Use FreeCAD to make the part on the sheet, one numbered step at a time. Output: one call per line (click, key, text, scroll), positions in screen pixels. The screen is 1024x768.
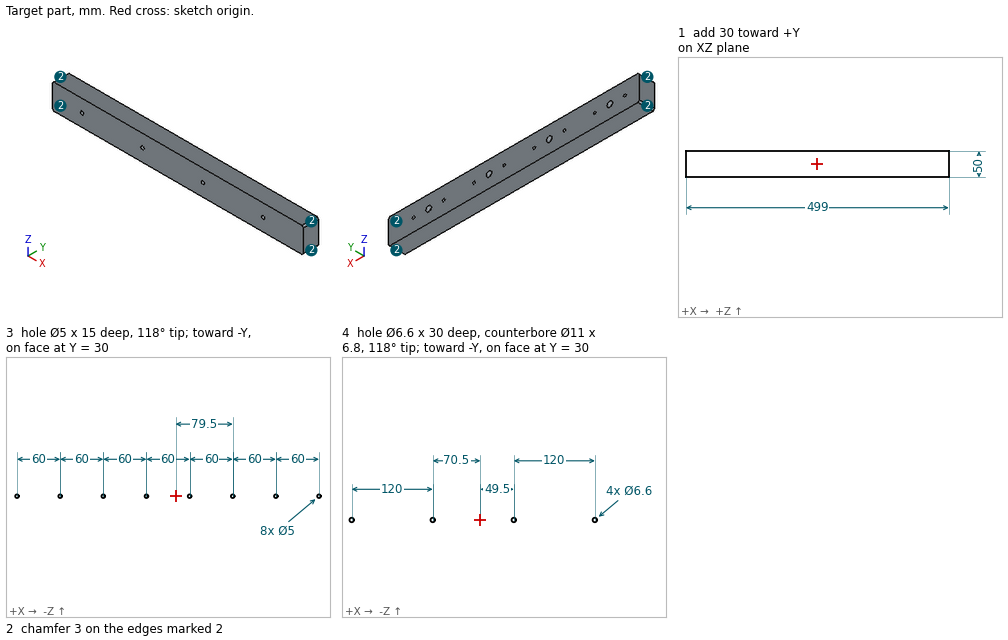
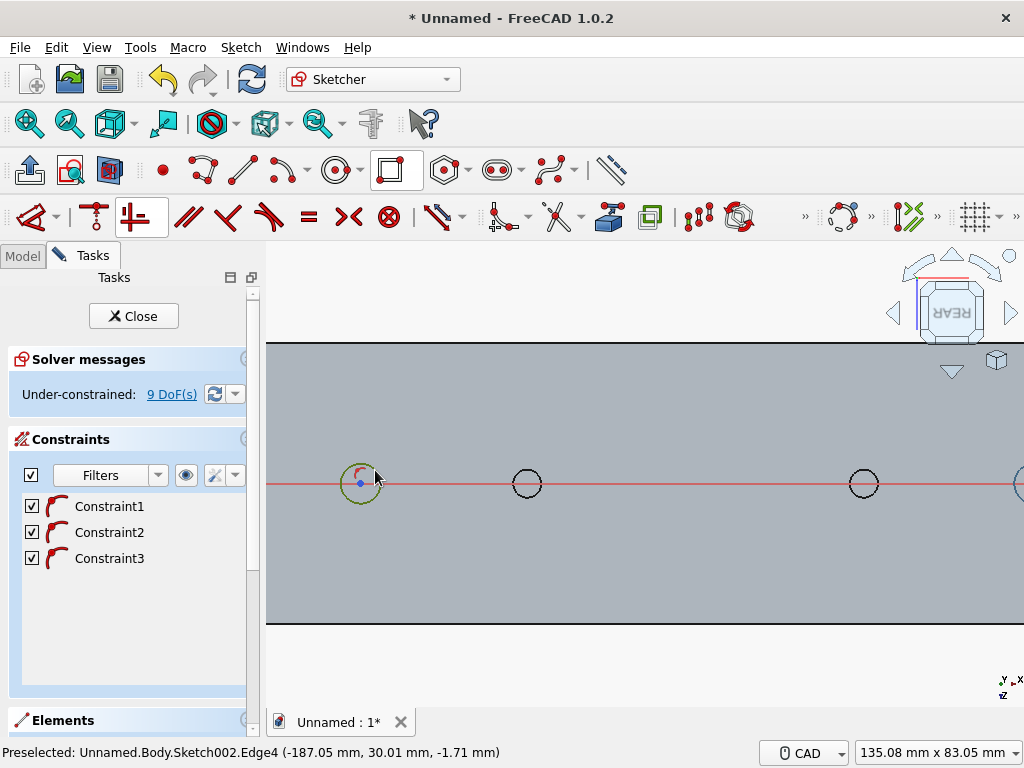
click(310, 218)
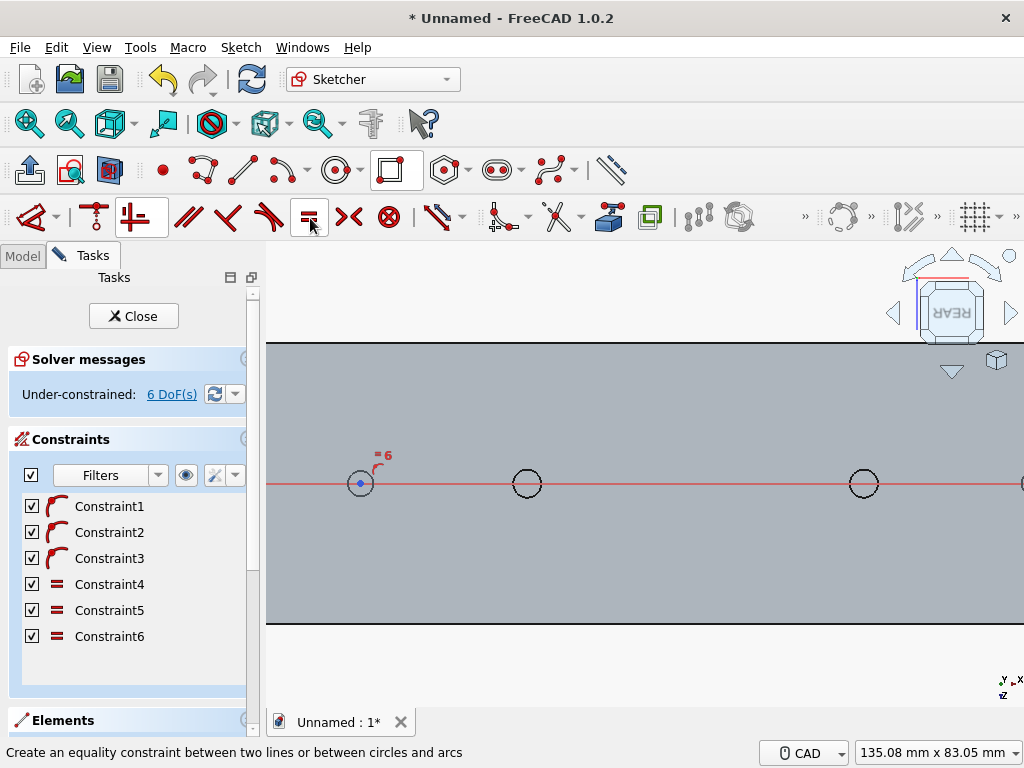
scroll(376, 472, down, 8)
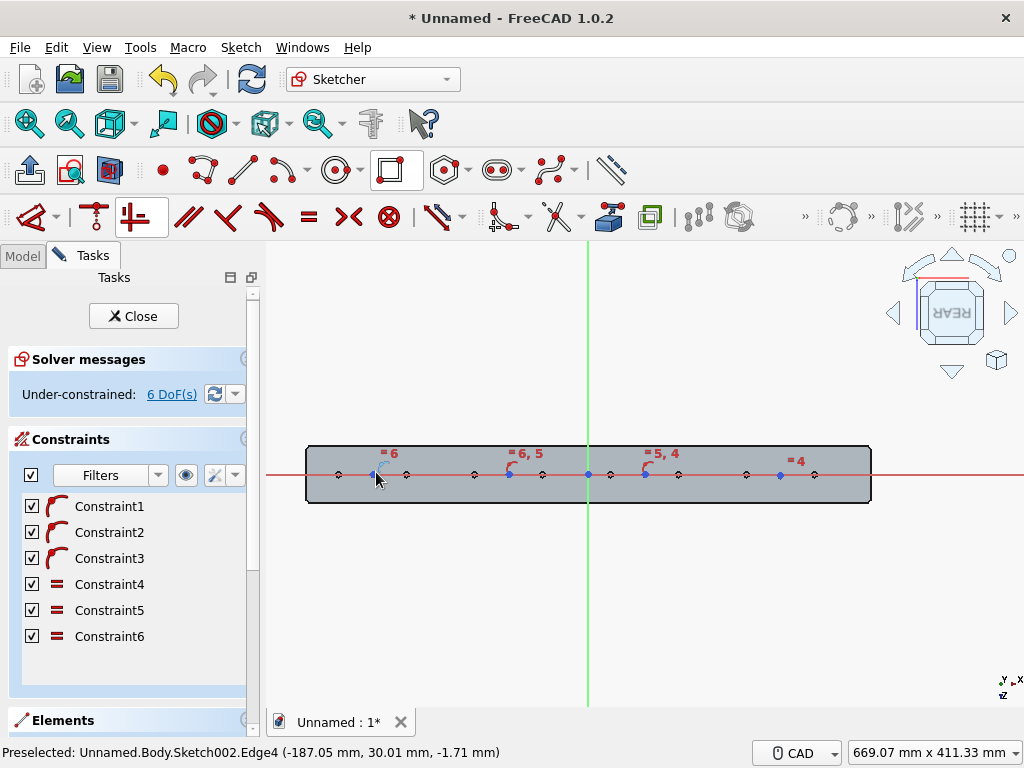
click(780, 476)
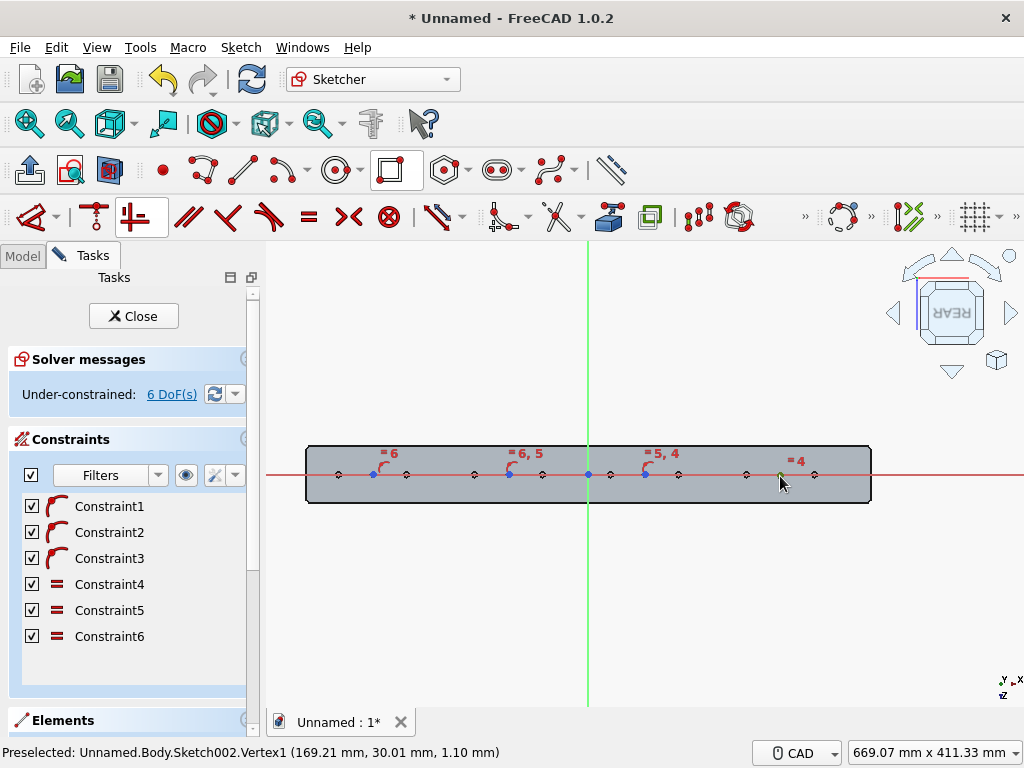
click(334, 475)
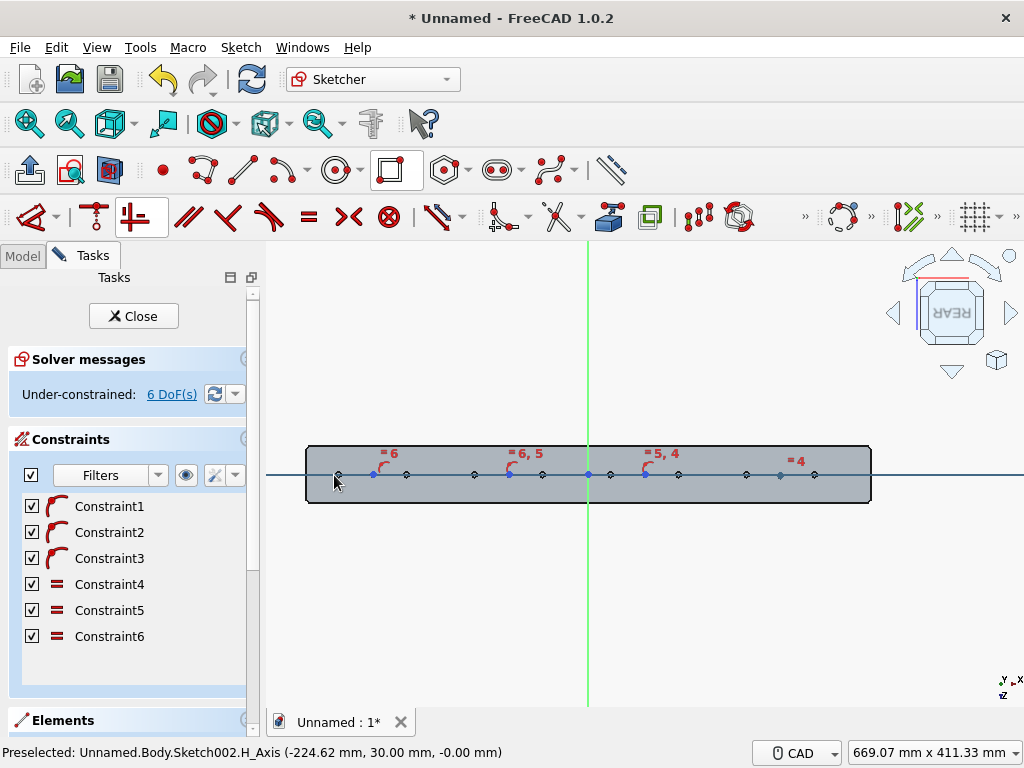
key(c)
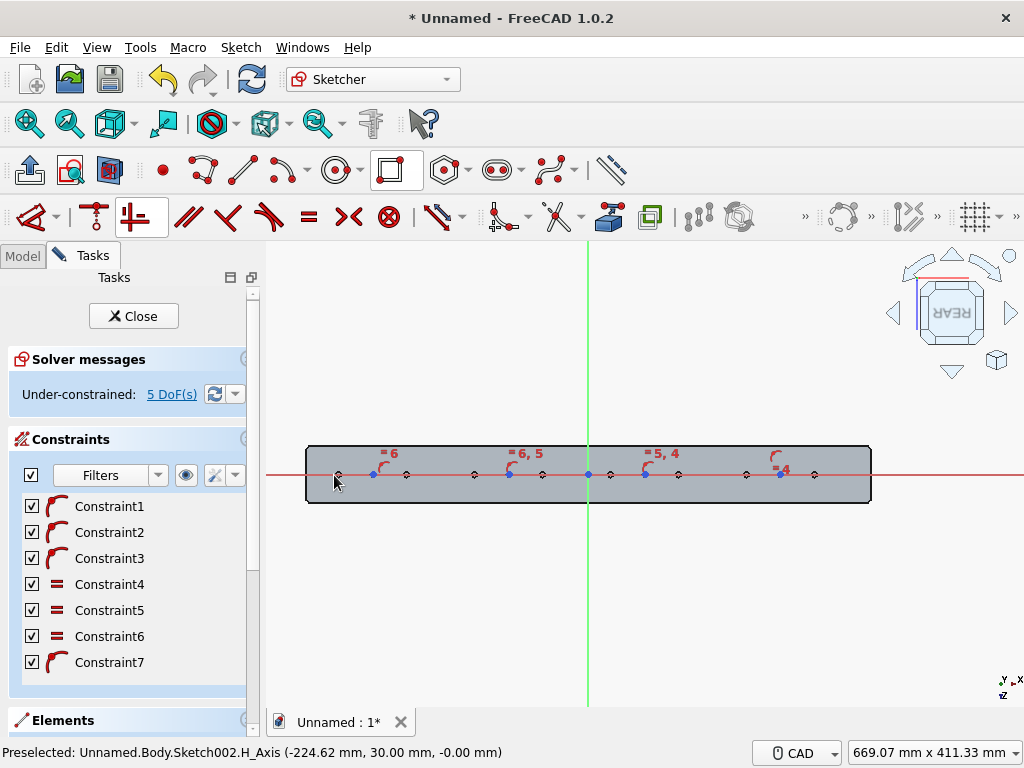
click(32, 218)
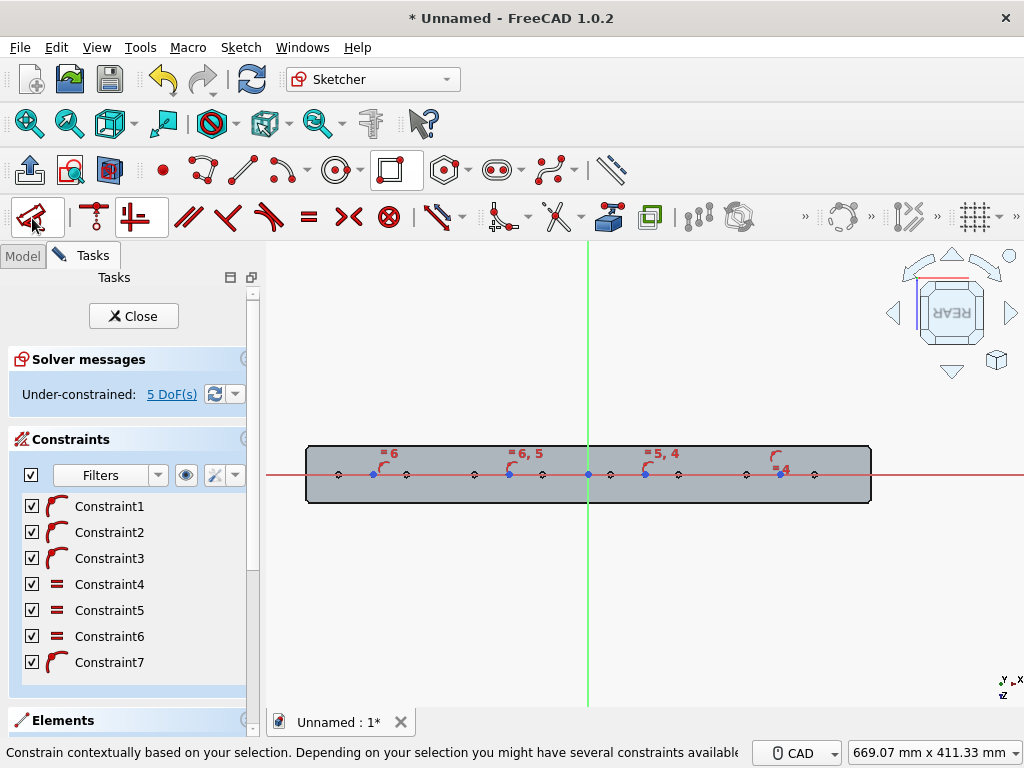
scroll(778, 477, up, 9)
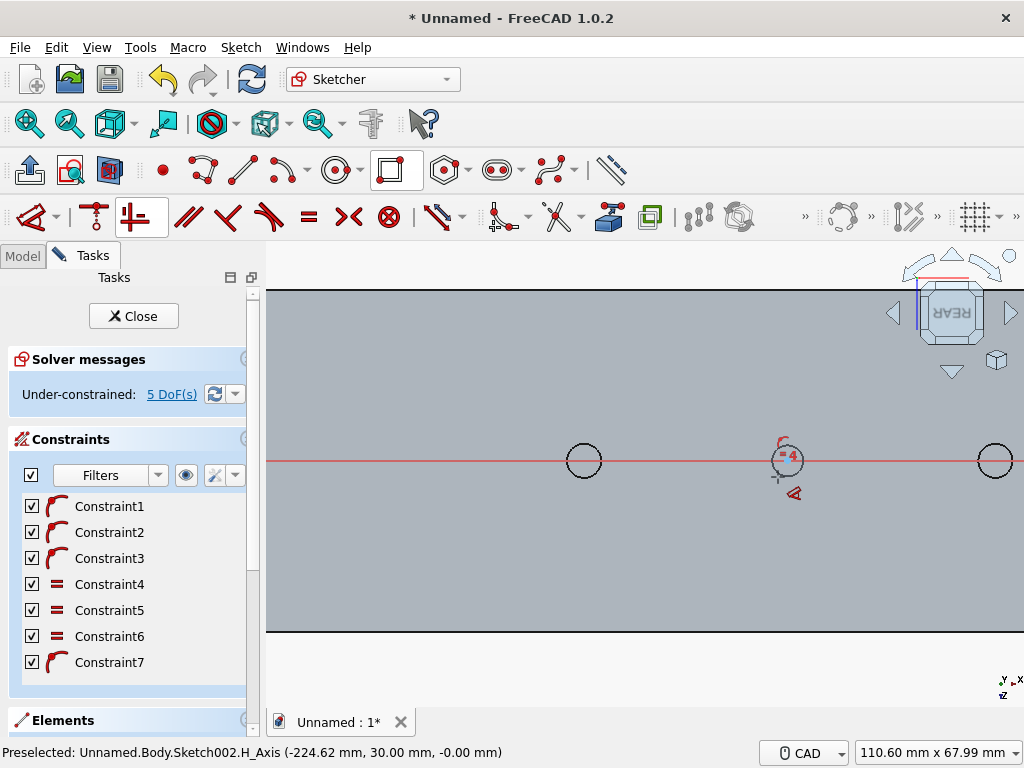
click(777, 472)
click(755, 495)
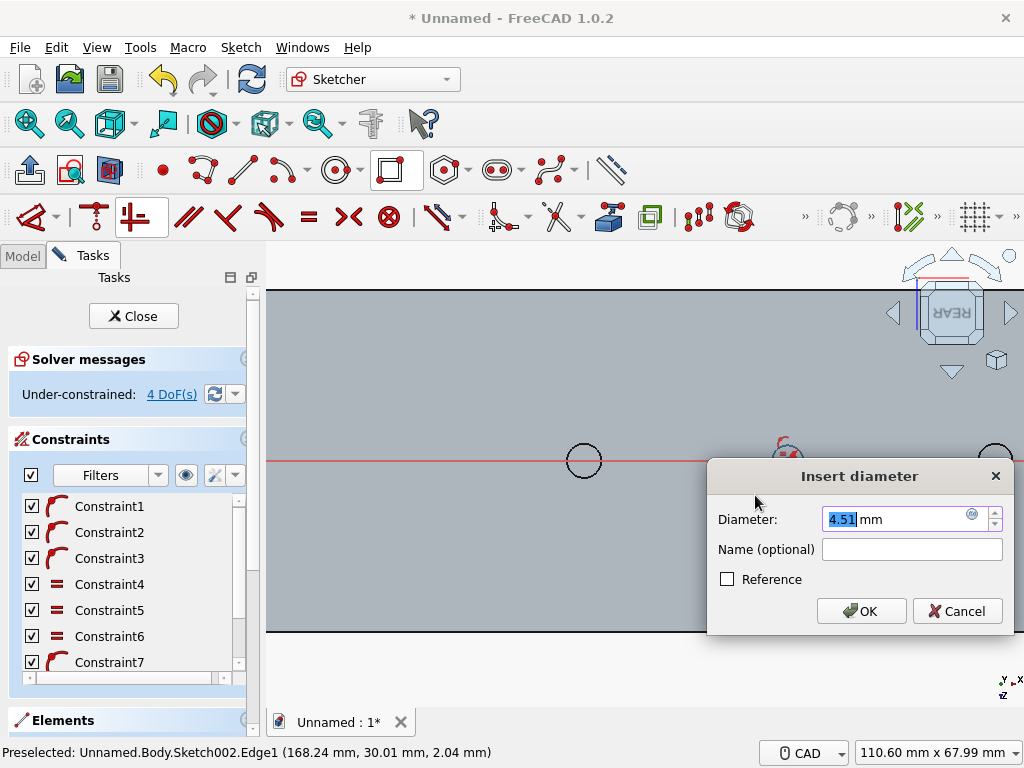
text(6.6)
key(Return)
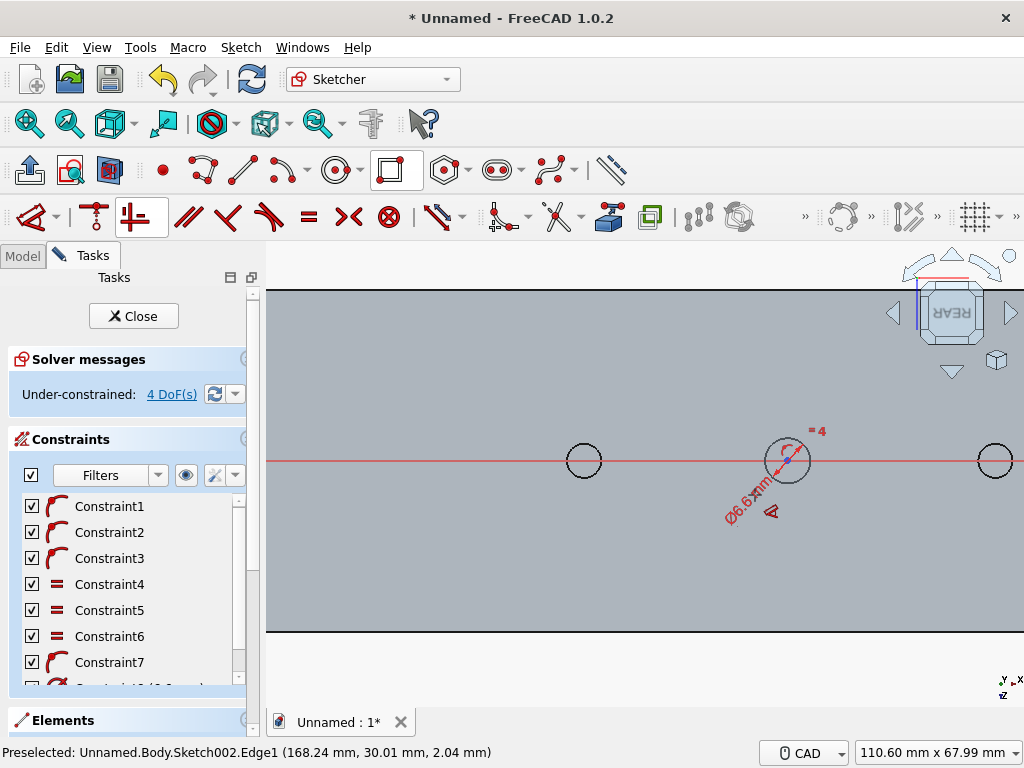
scroll(779, 477, down, 9)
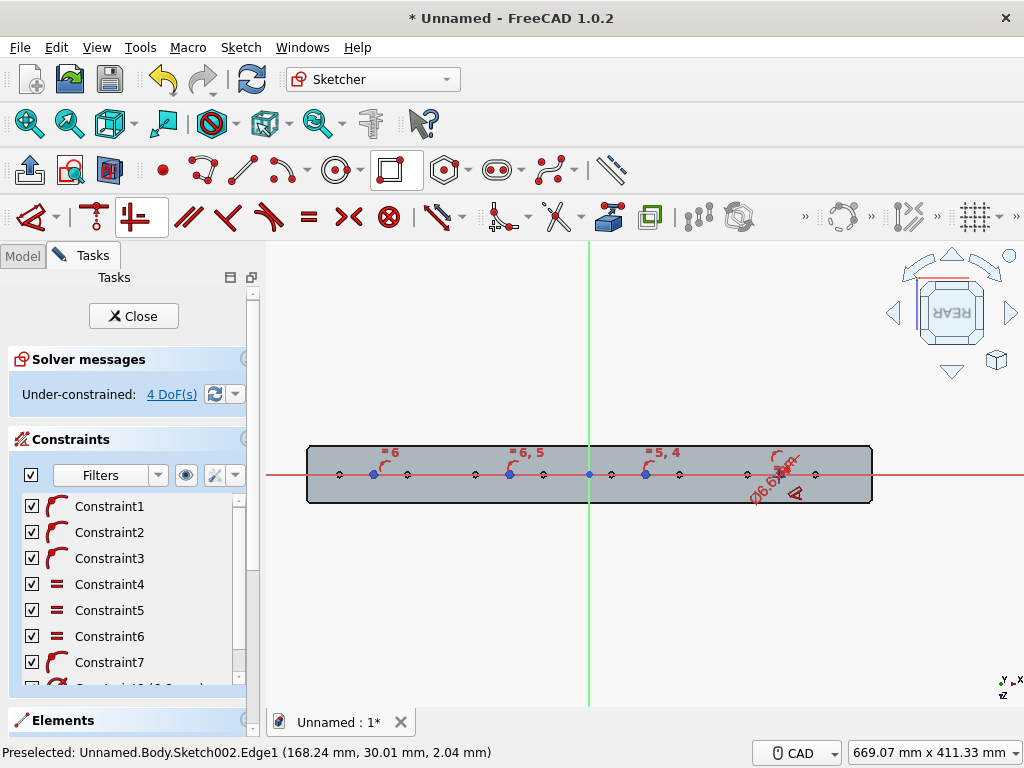
click(646, 475)
click(618, 509)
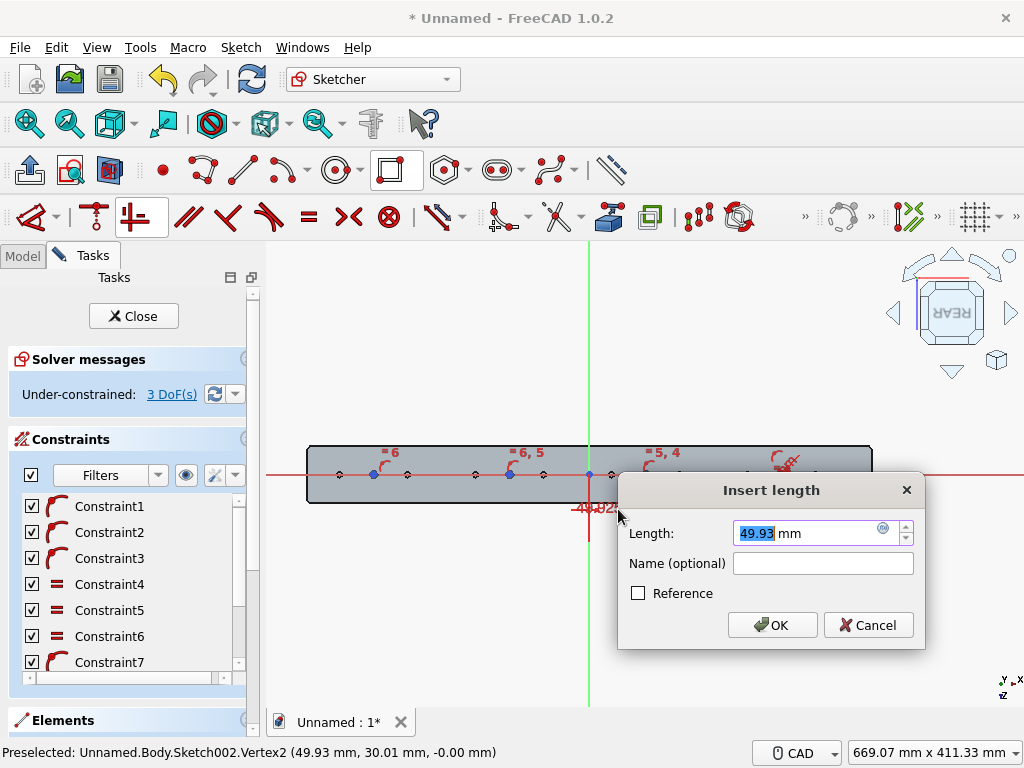
text(49.5)
key(Return)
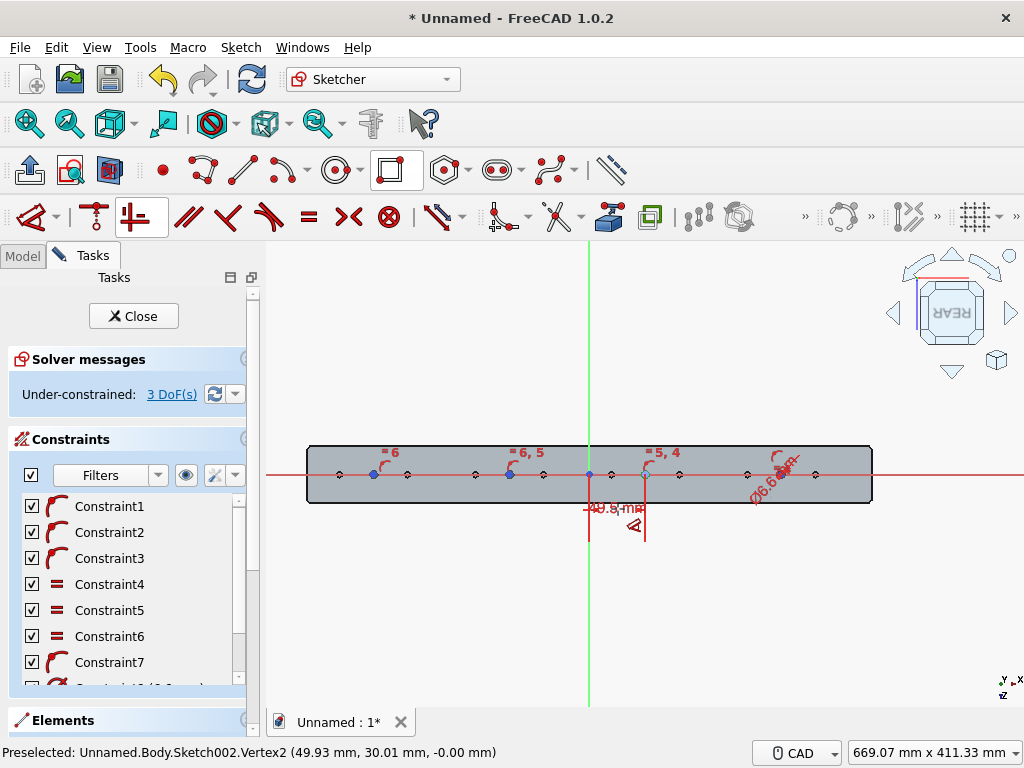
click(510, 475)
click(531, 509)